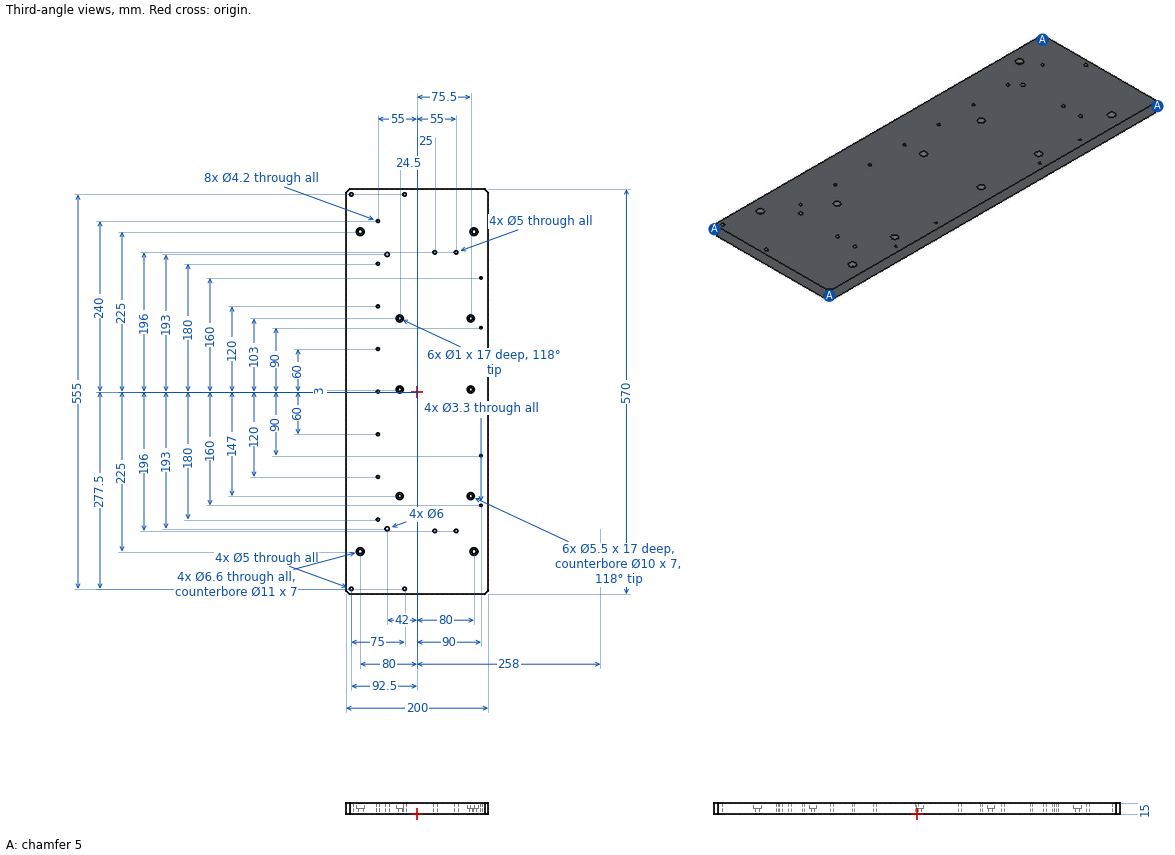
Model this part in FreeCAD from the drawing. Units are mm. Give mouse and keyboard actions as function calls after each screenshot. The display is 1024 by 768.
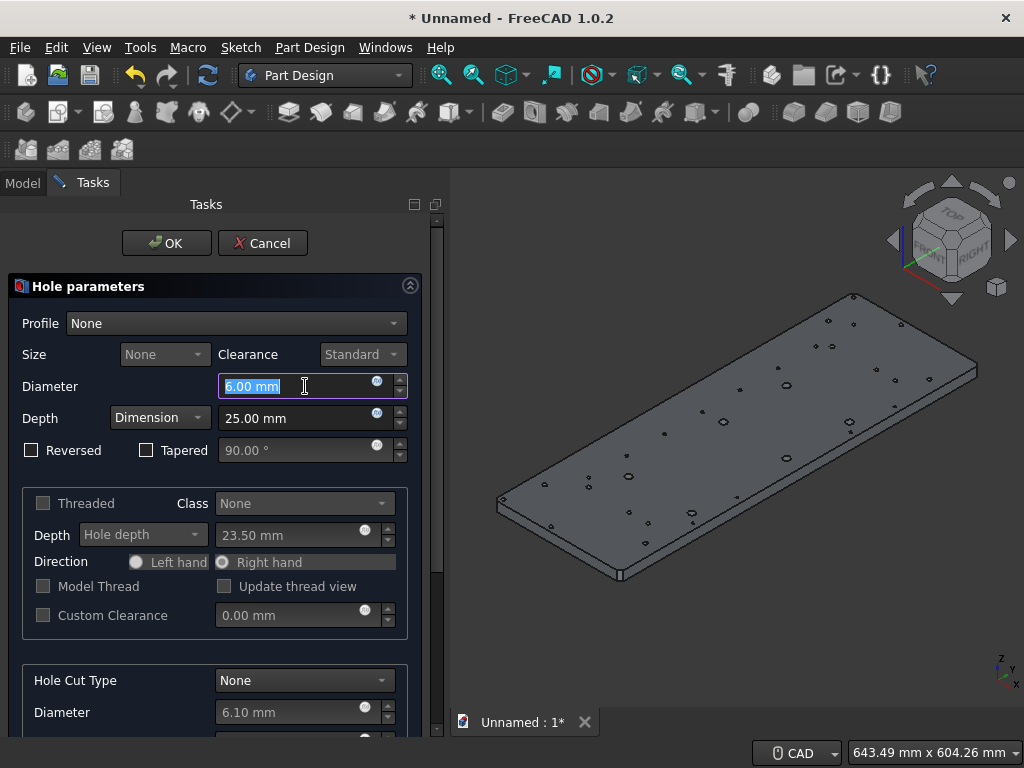
text(6.6)
key(Tab)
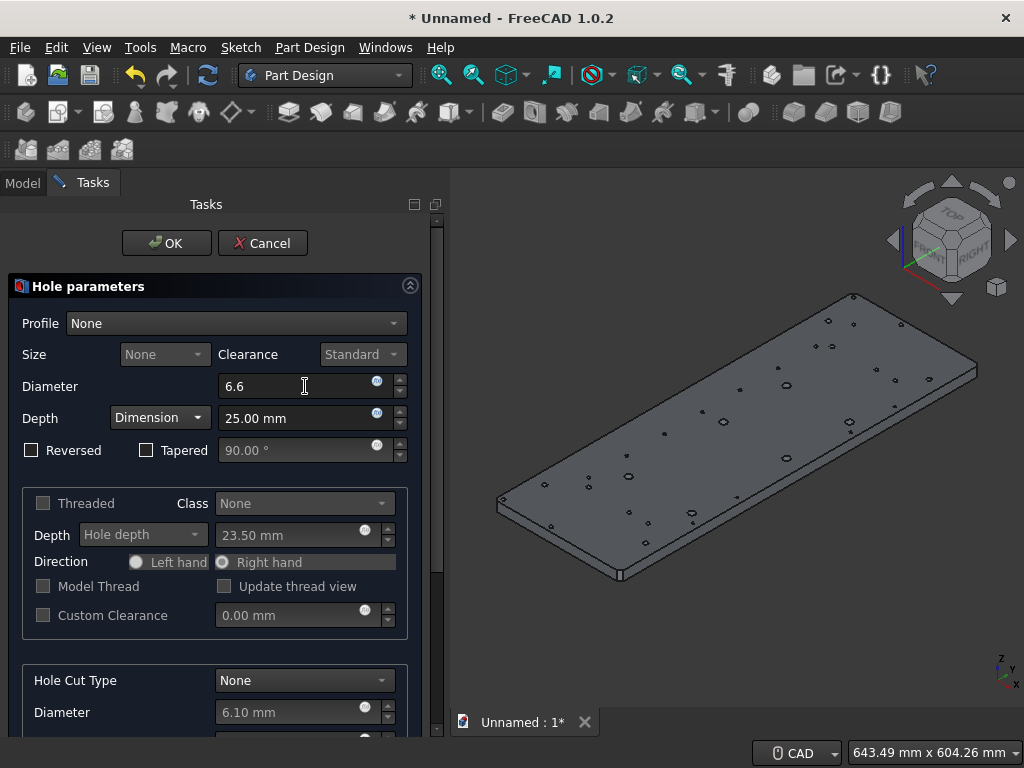
click(161, 418)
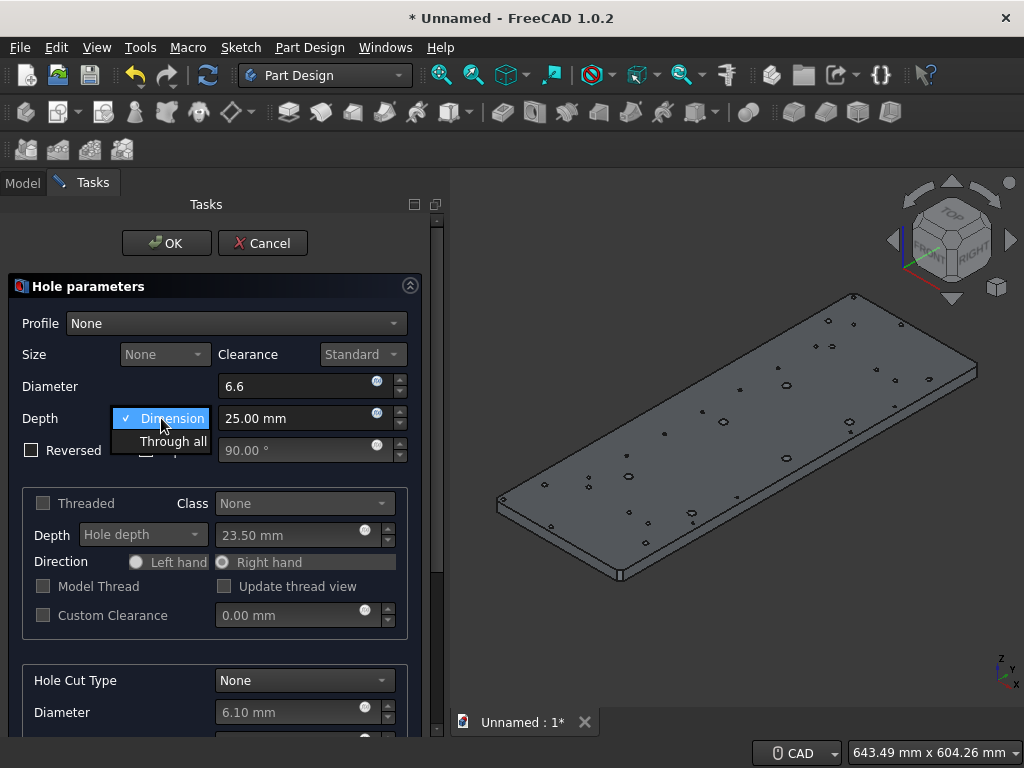
click(160, 442)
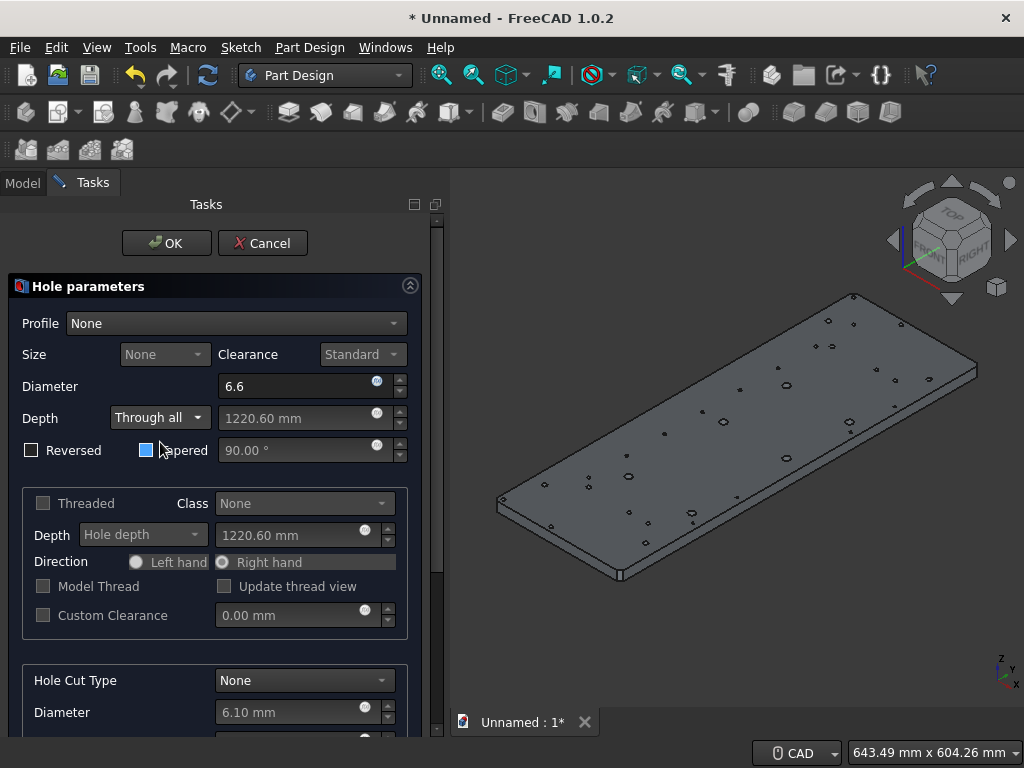
click(306, 680)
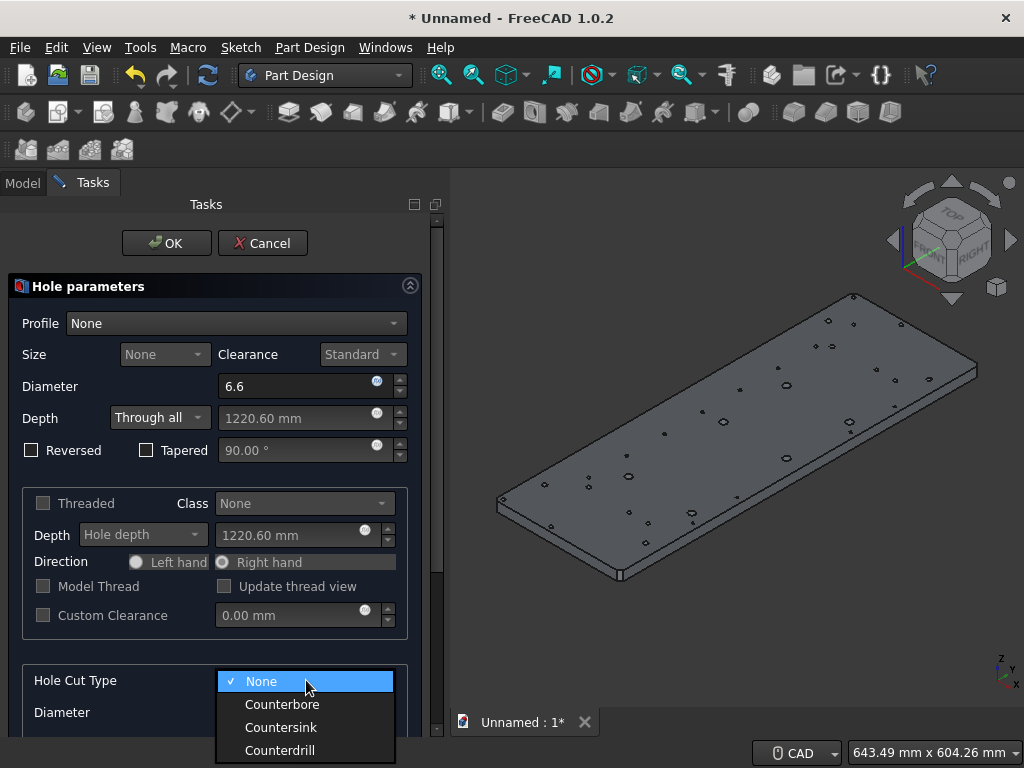
click(304, 704)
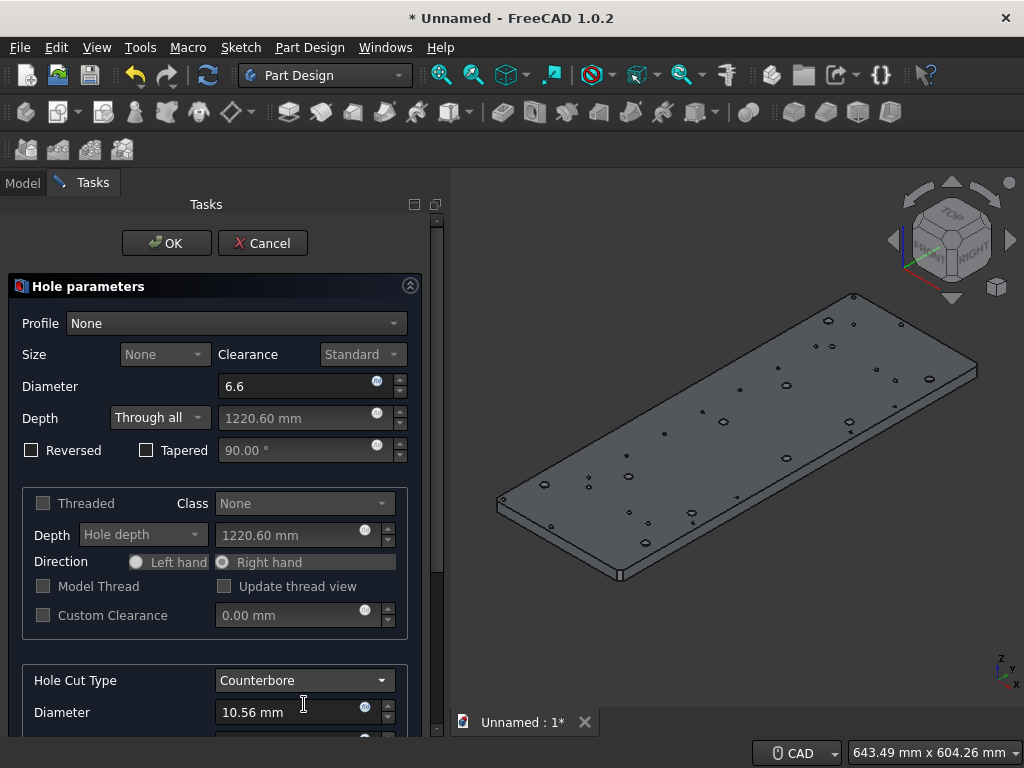
triple_click(298, 712)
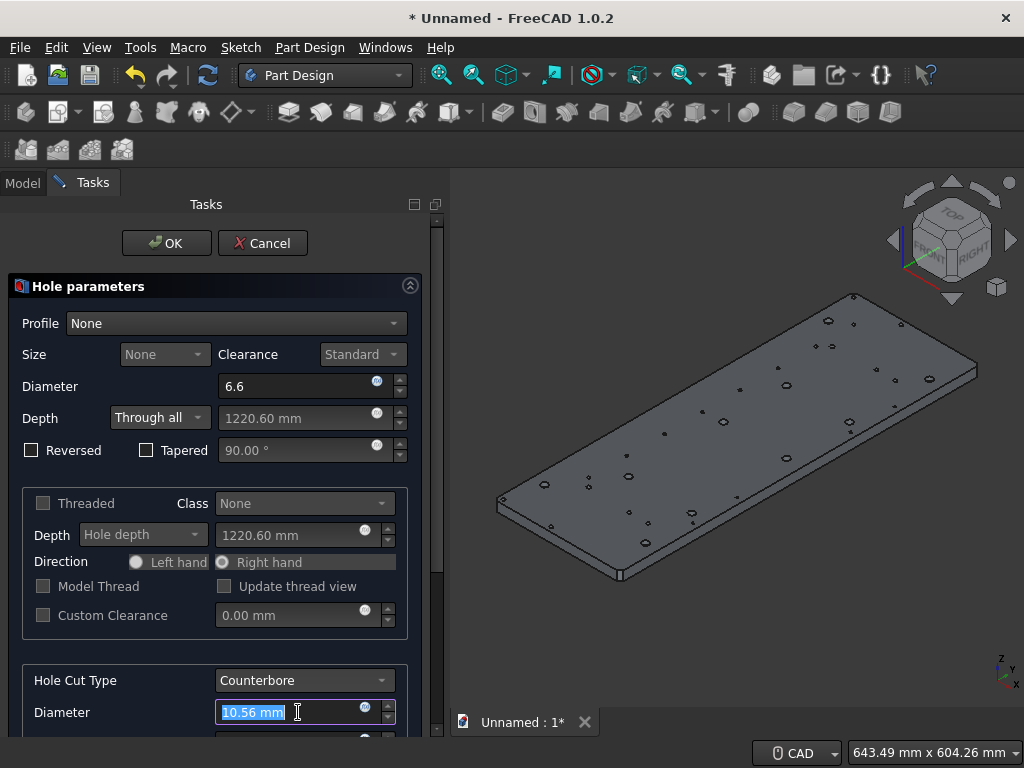
text(11)
key(Tab)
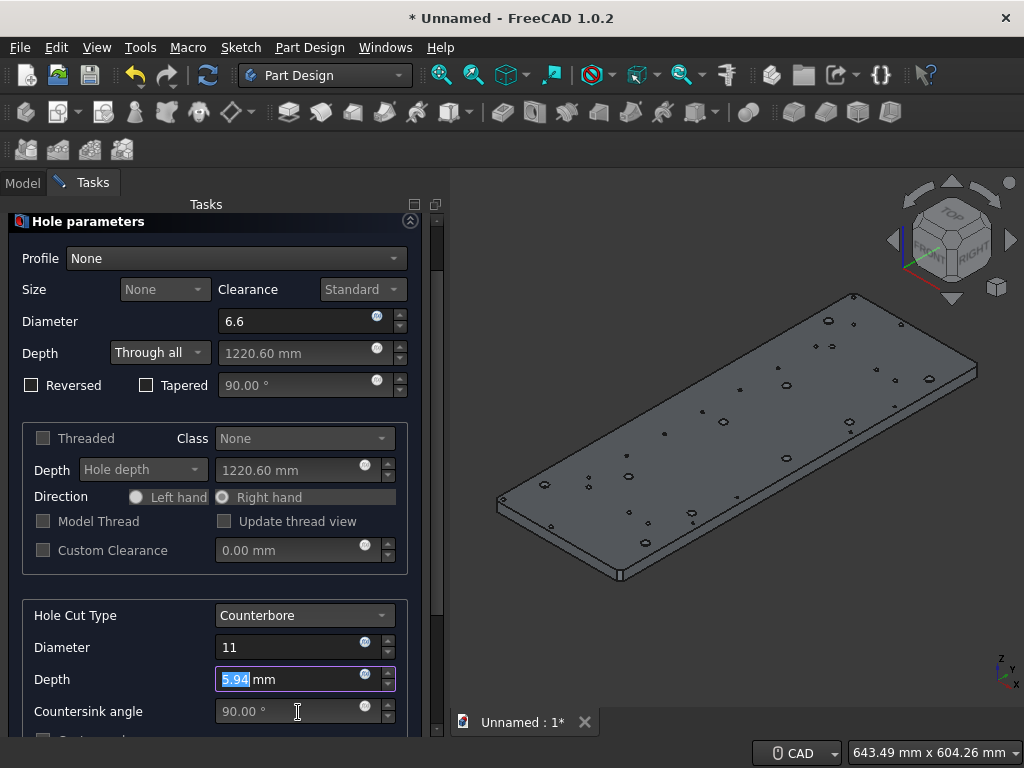
text(7)
key(Tab)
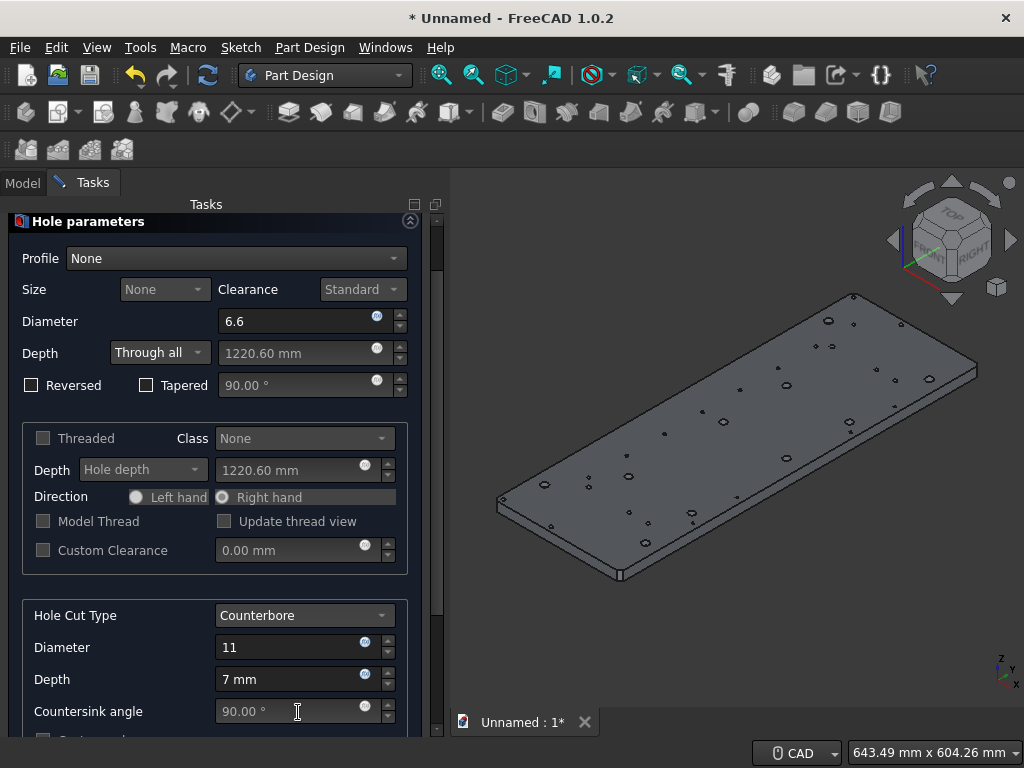
scroll(437, 475, up, 2)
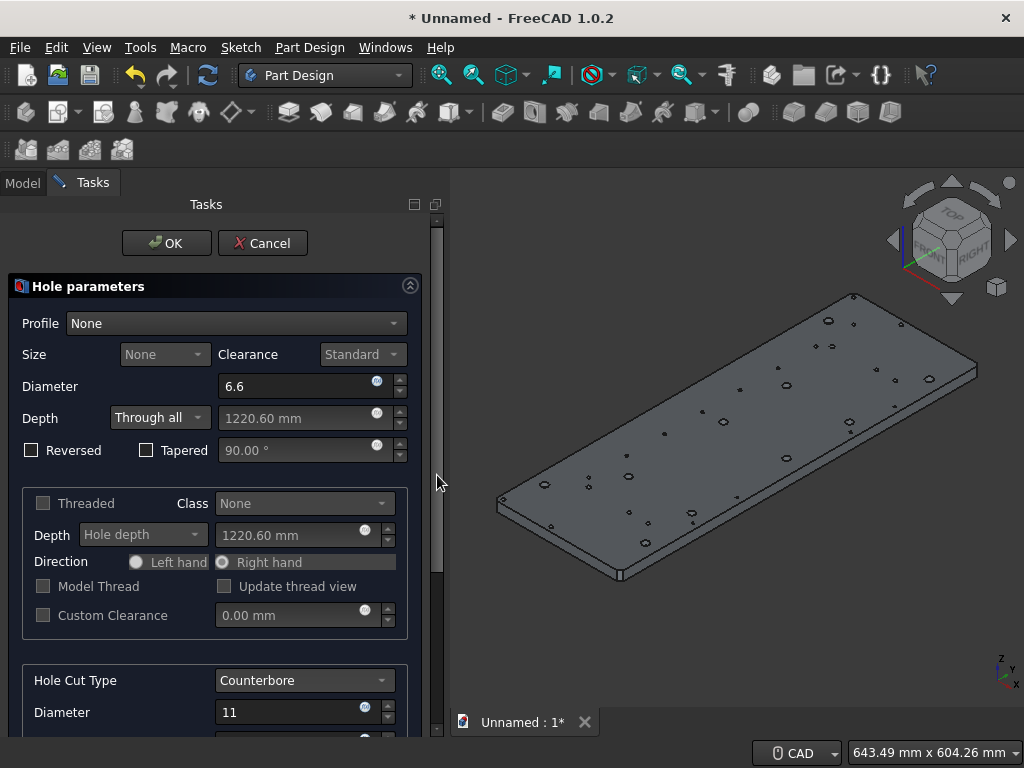
click(167, 243)